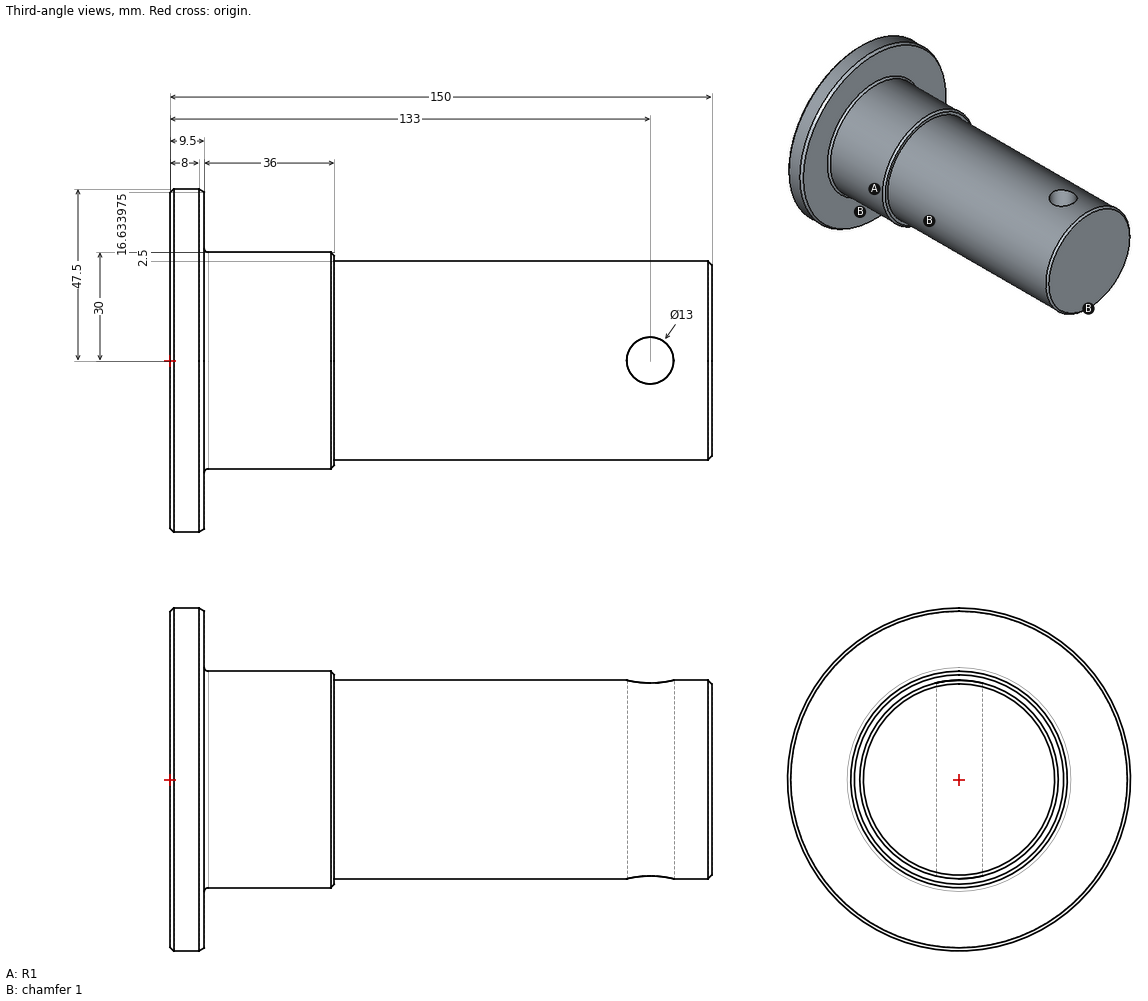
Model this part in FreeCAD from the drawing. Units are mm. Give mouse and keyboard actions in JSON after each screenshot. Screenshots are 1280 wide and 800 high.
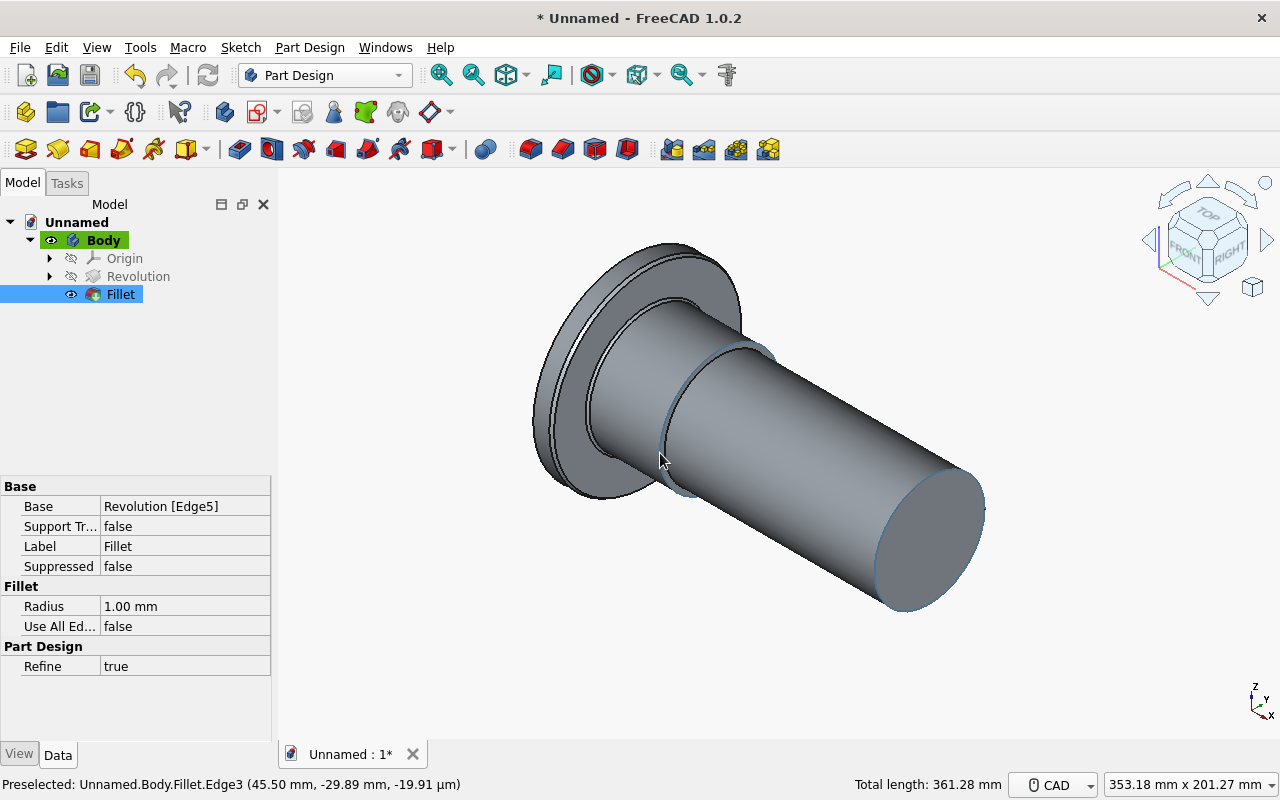
{"action": "left_click", "coordinate": [599, 278], "text": "ctrl"}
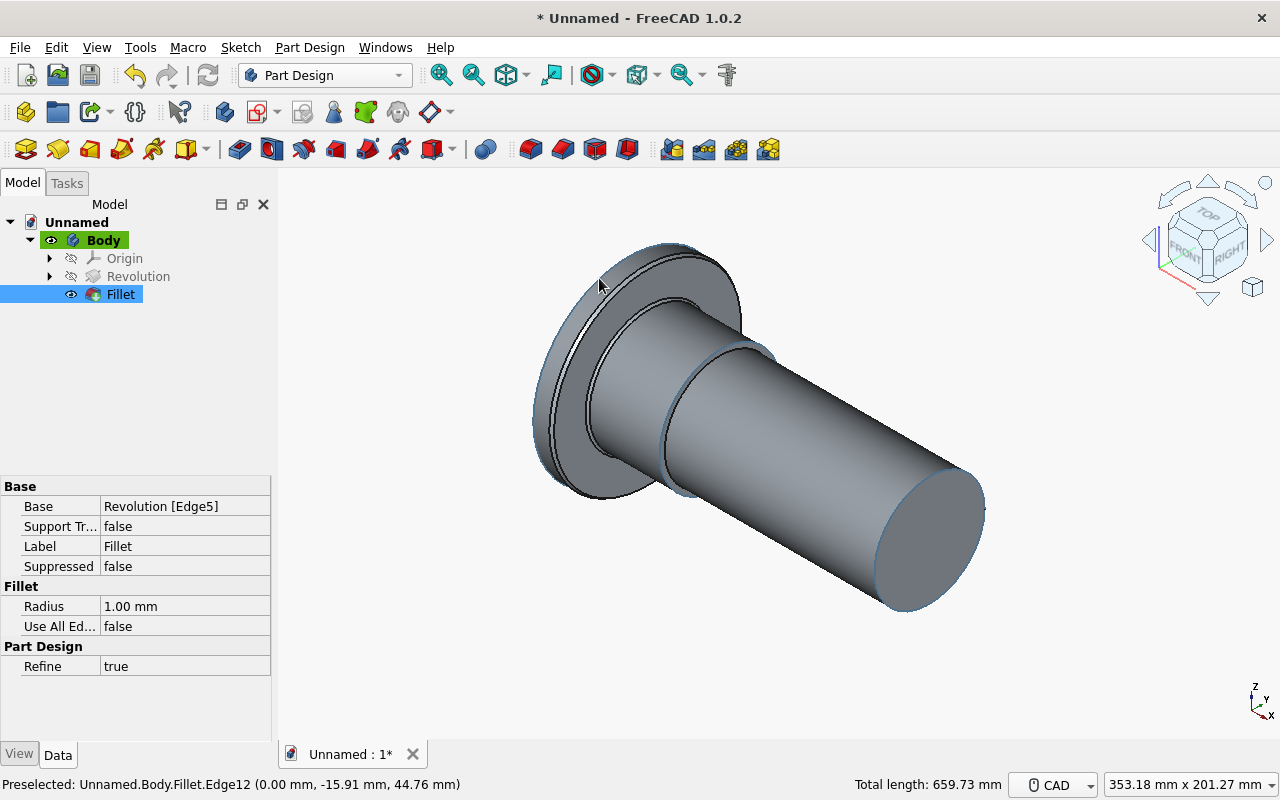
{"action": "left_click", "coordinate": [564, 150]}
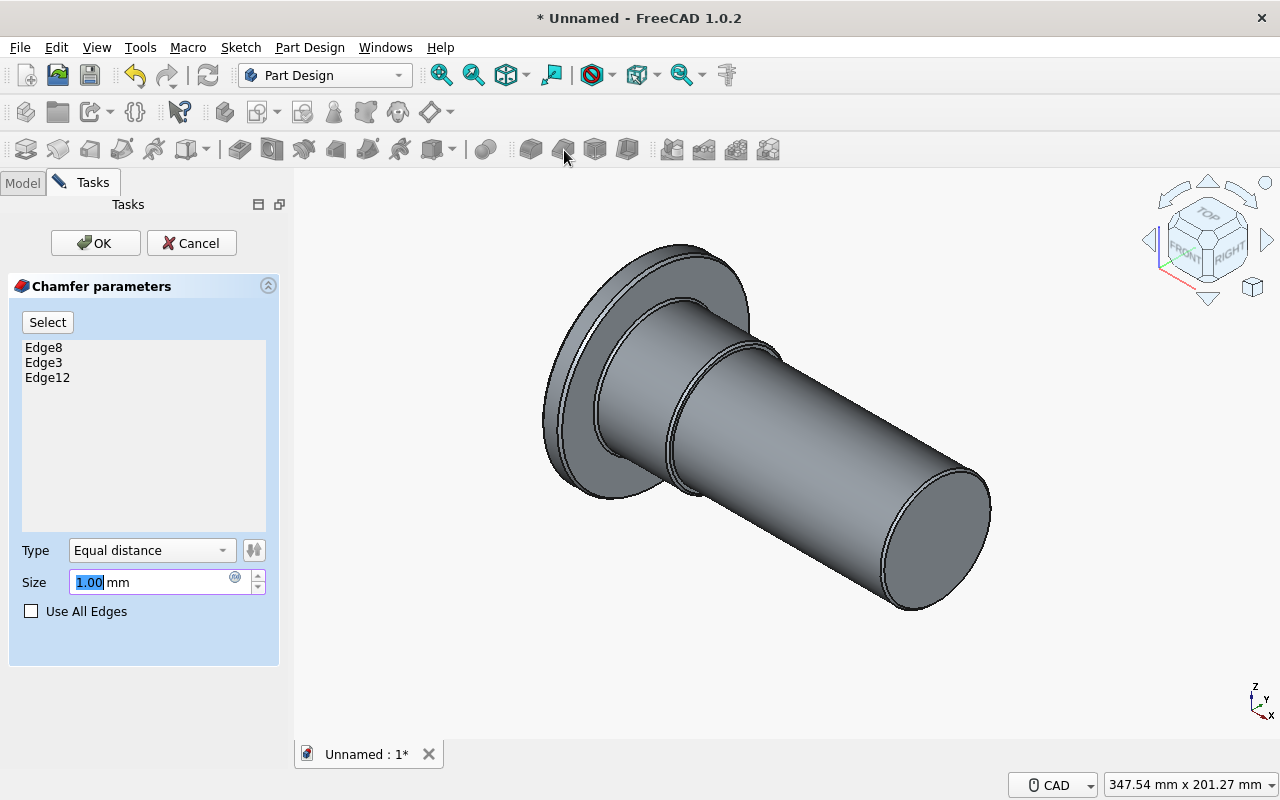
{"action": "type", "text": "1"}
{"action": "key", "text": "Tab"}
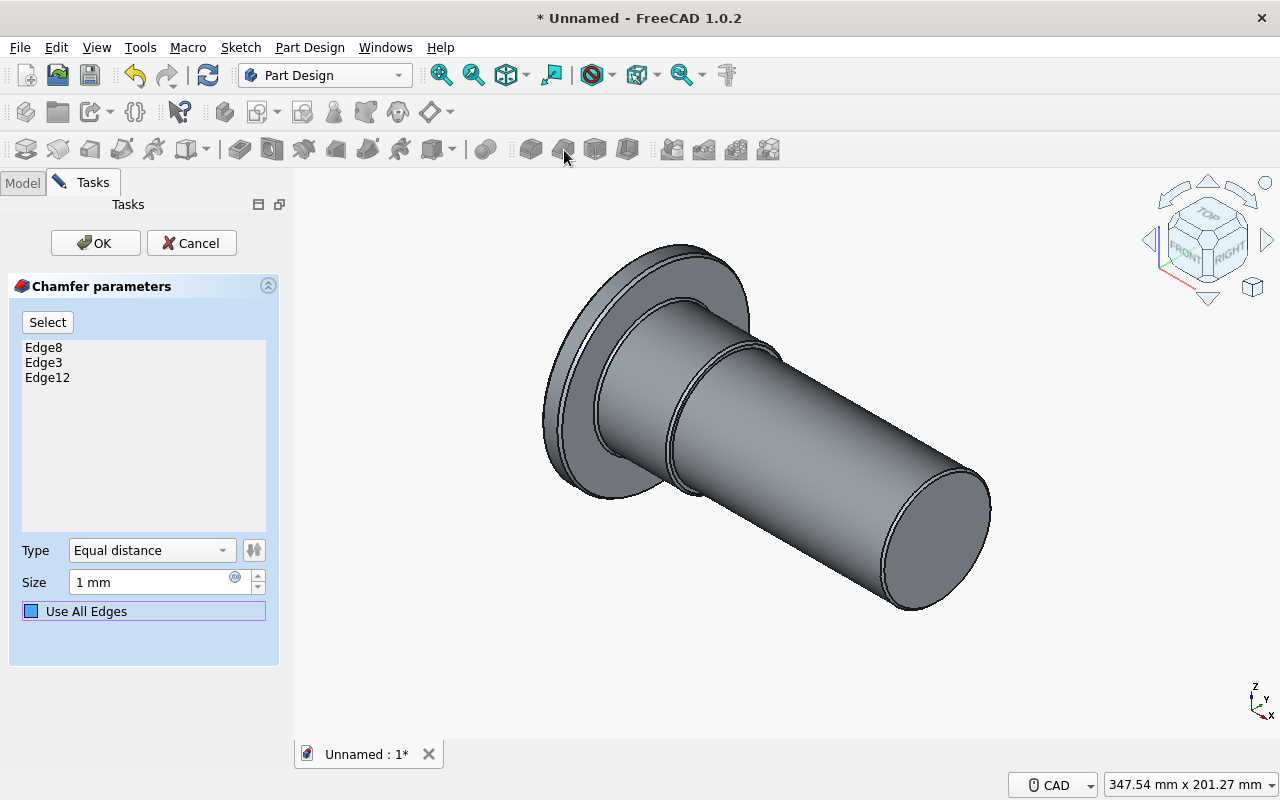
{"action": "left_click", "coordinate": [96, 243]}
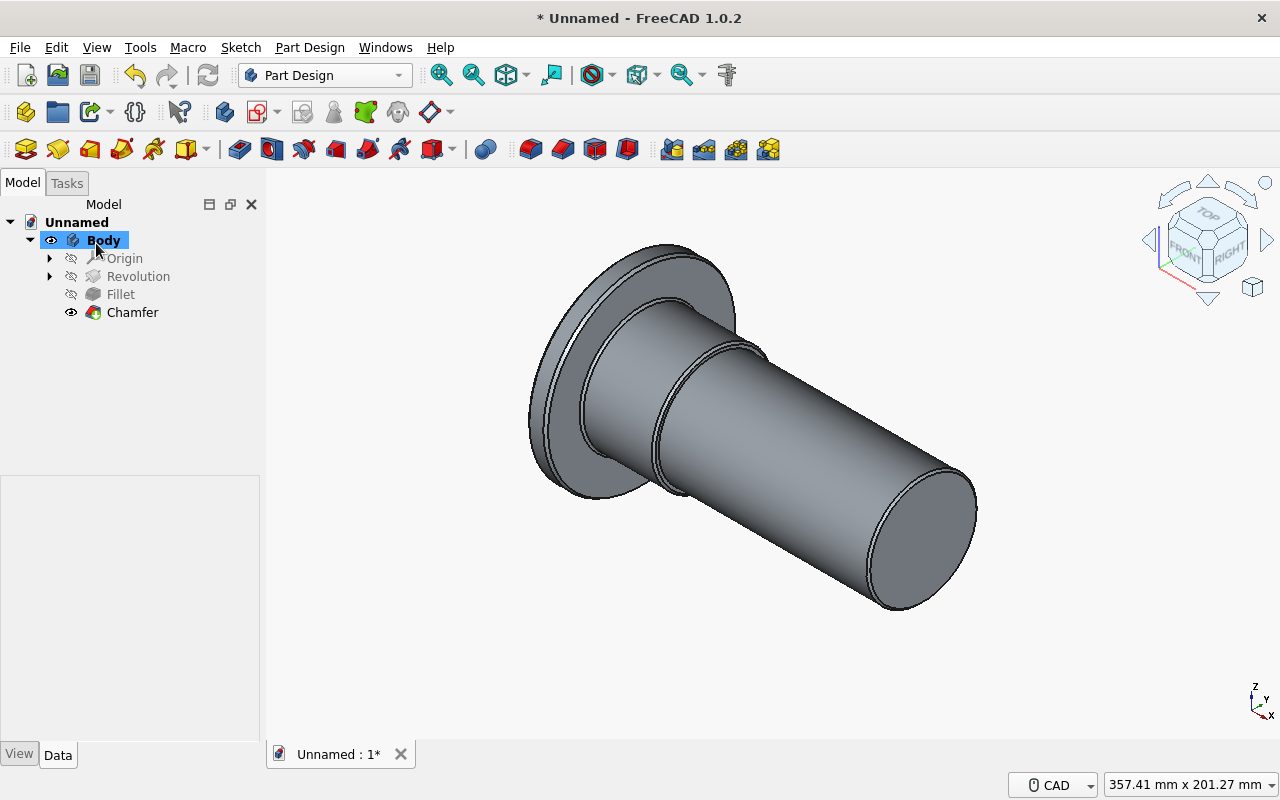
{"action": "left_click", "coordinate": [258, 112]}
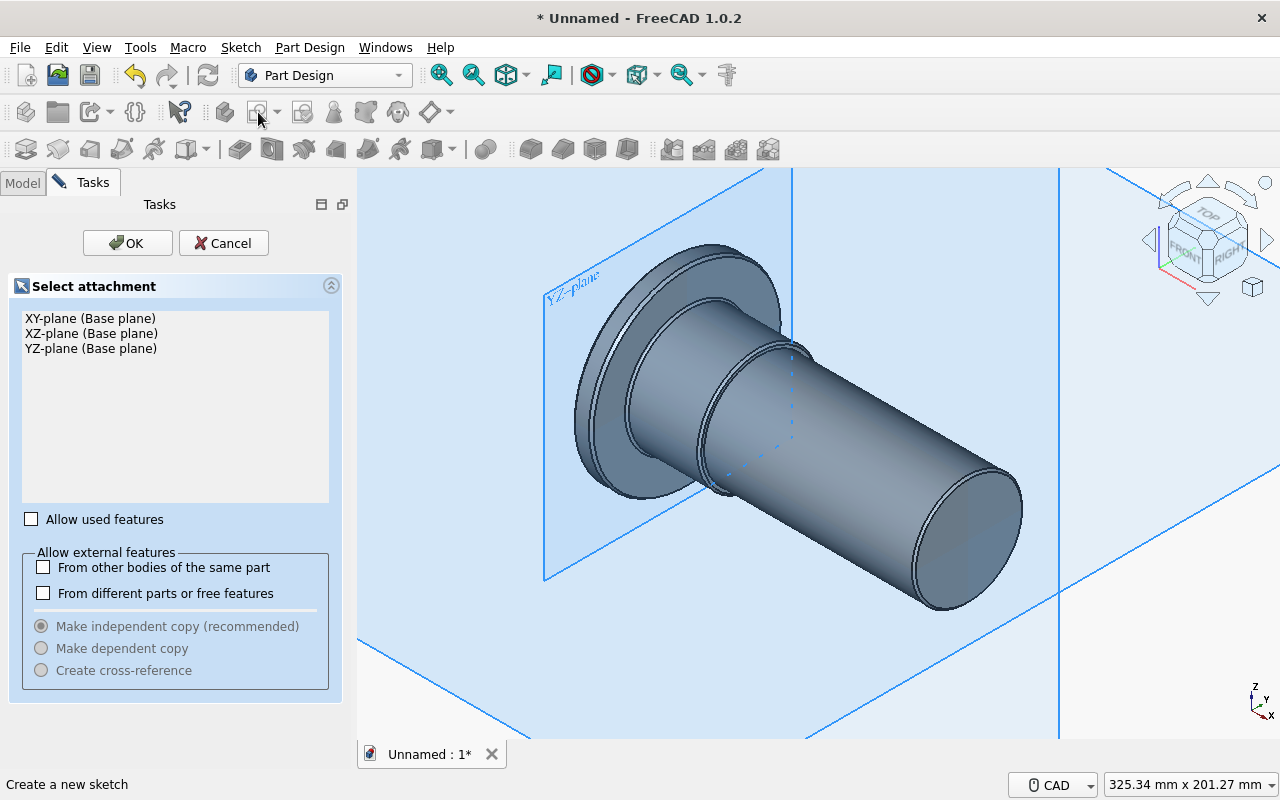
{"action": "left_click", "coordinate": [82, 318]}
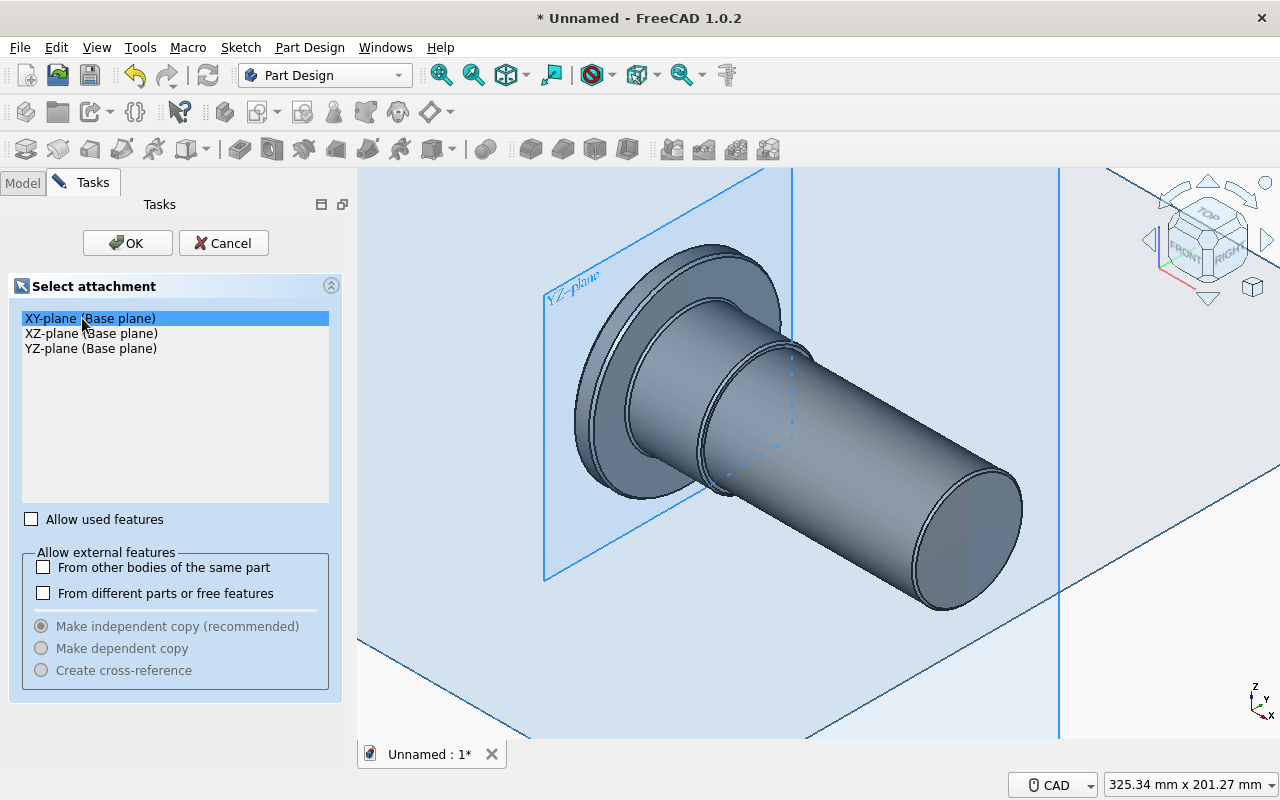
{"action": "left_click", "coordinate": [128, 243]}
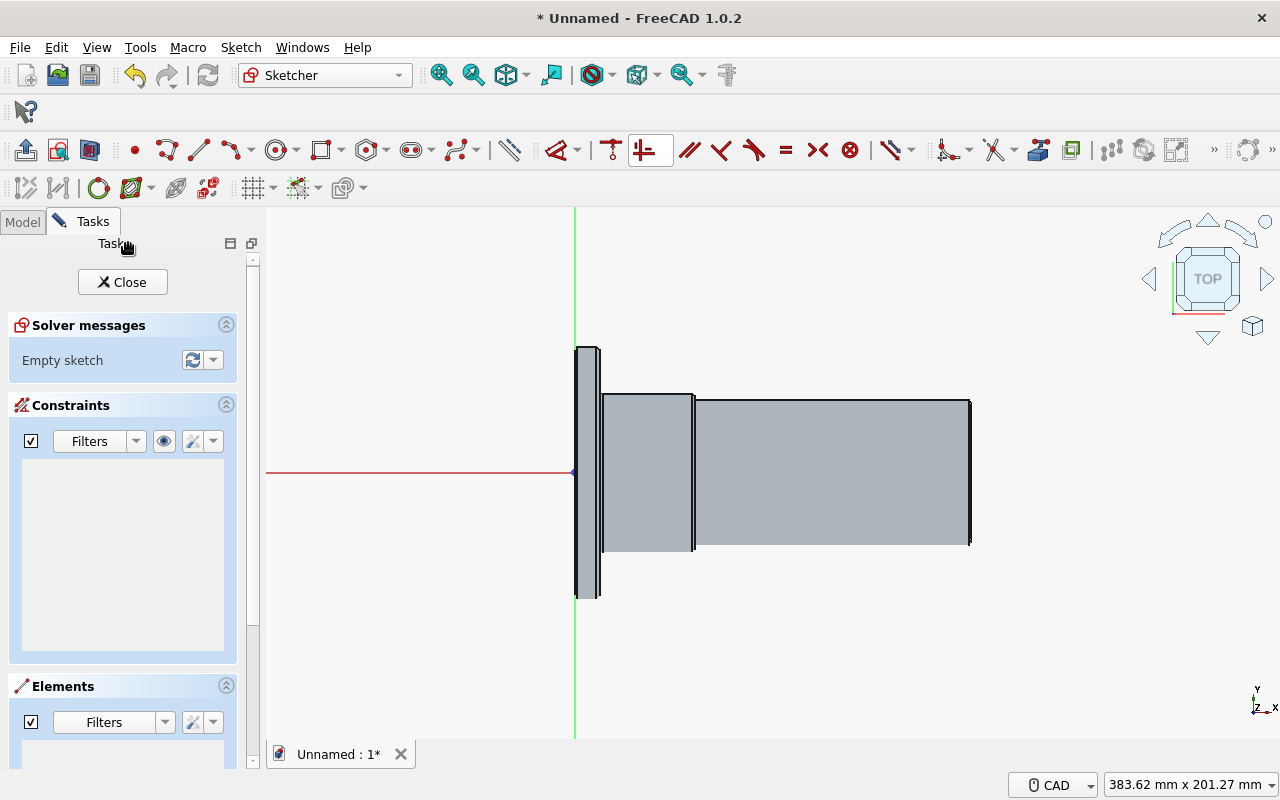
{"action": "left_click", "coordinate": [90, 150]}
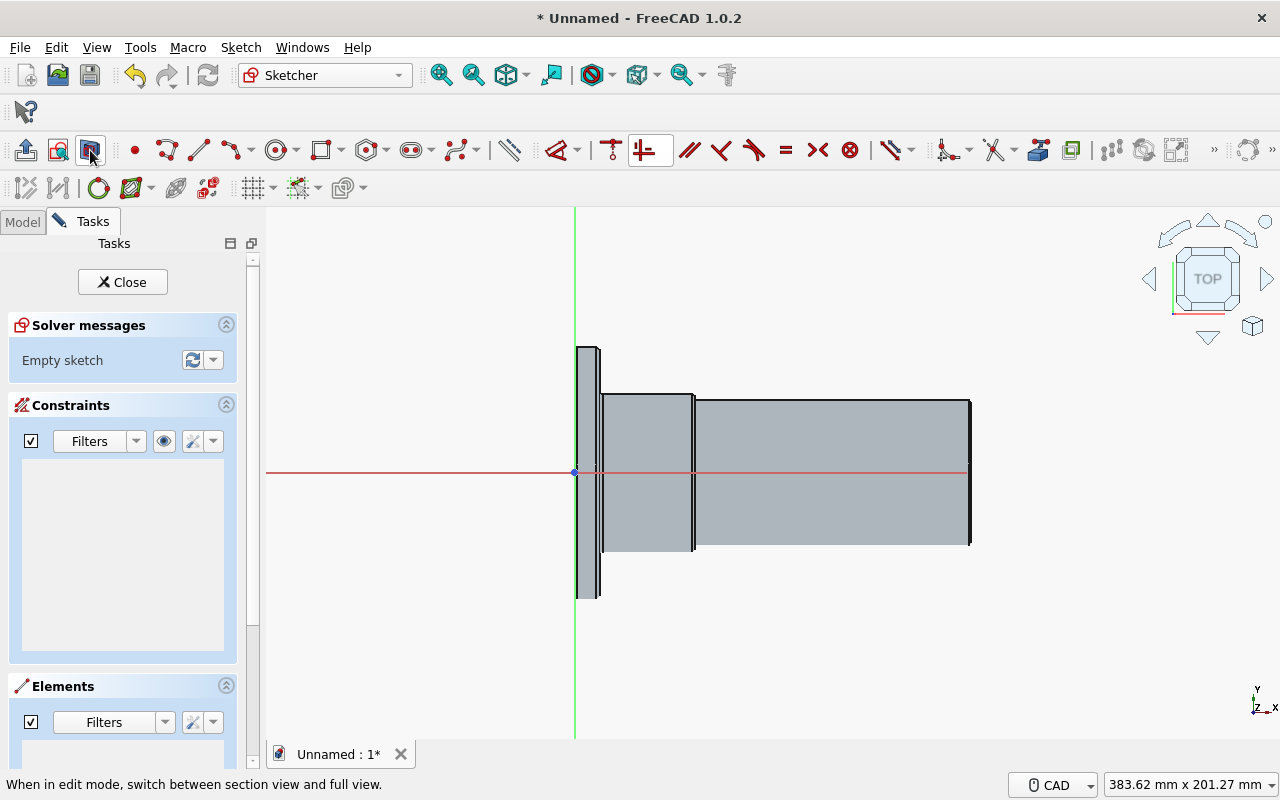
{"action": "scroll", "coordinate": [954, 473], "scroll_direction": "up", "scroll_amount": 11}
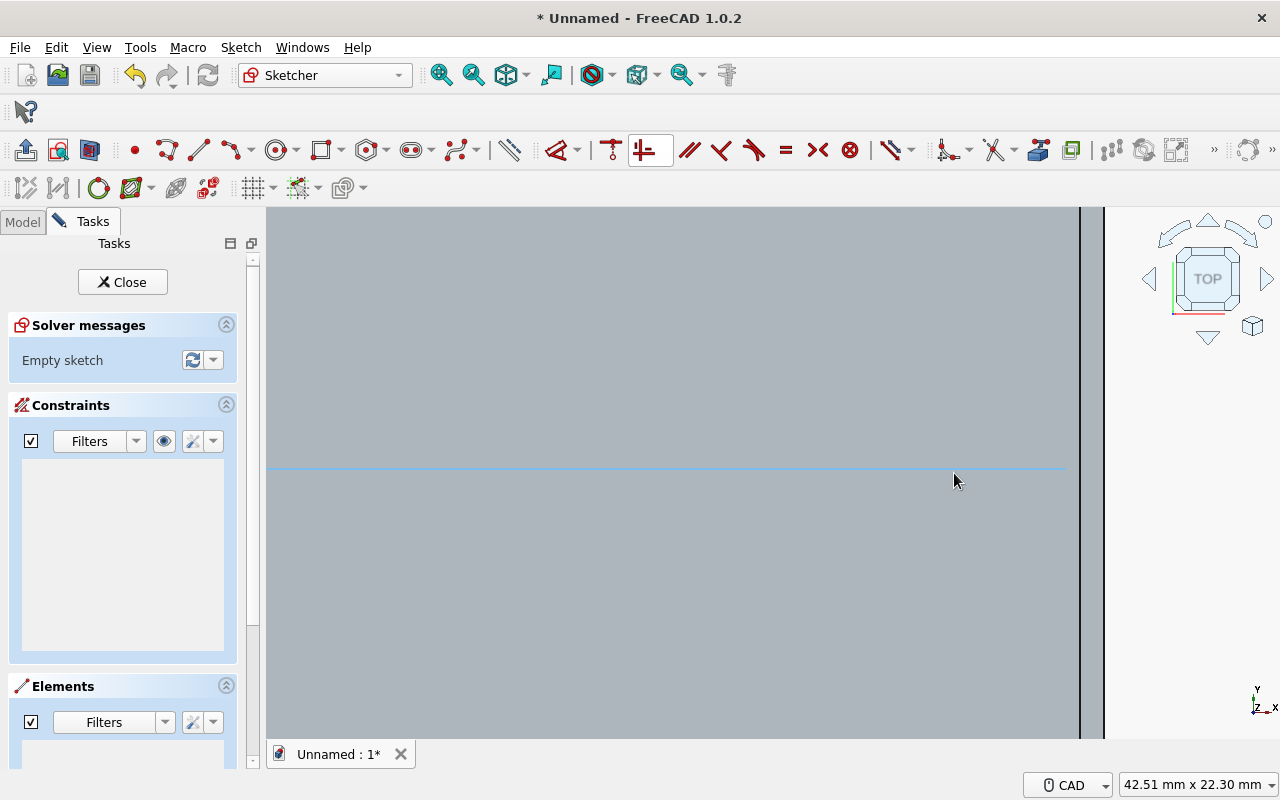
{"action": "key", "text": "g c"}